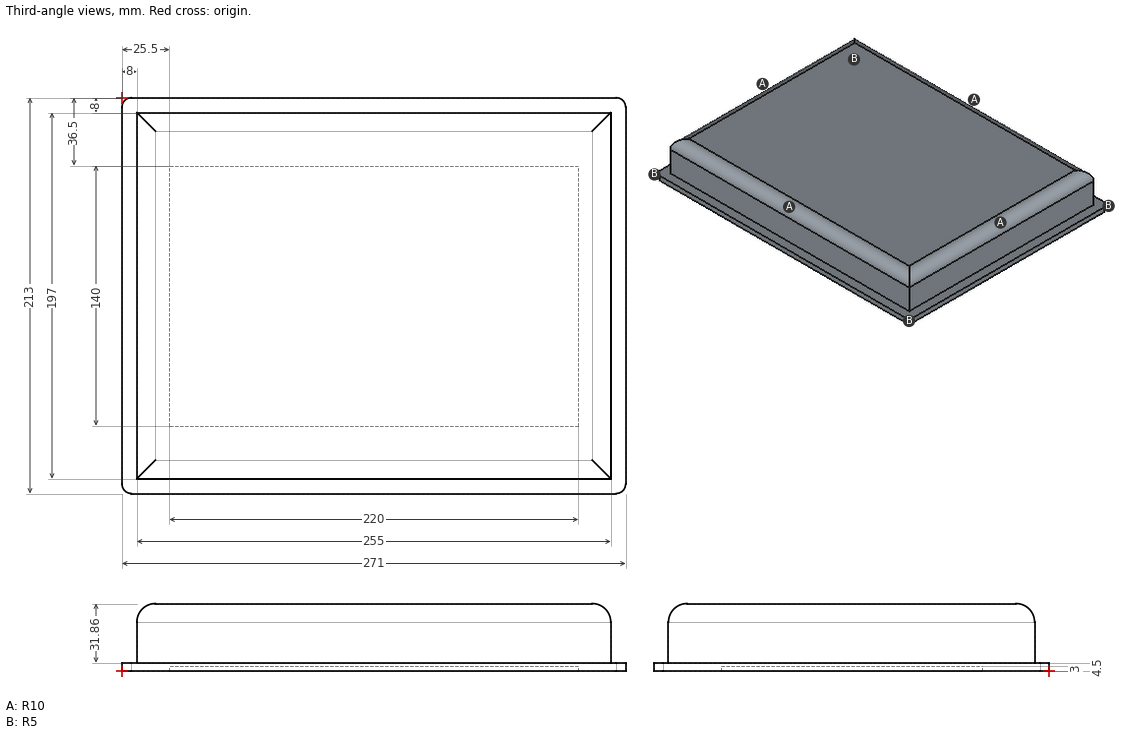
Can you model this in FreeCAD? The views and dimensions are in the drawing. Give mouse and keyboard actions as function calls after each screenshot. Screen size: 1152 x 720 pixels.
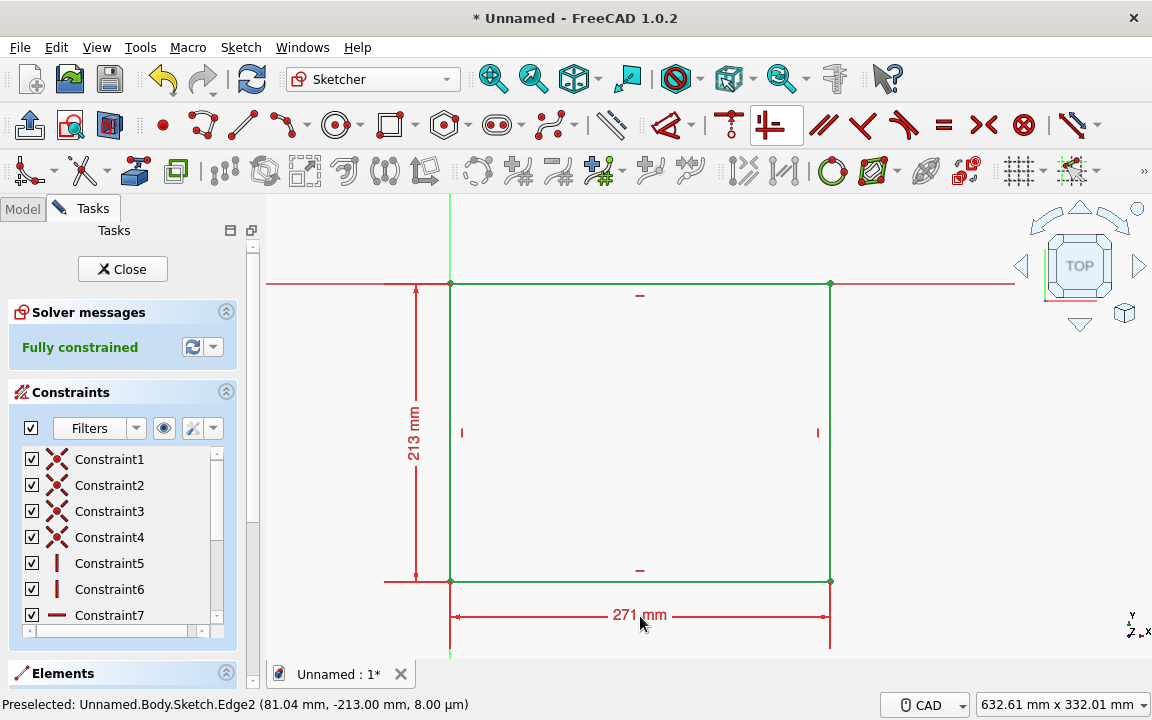
click(123, 269)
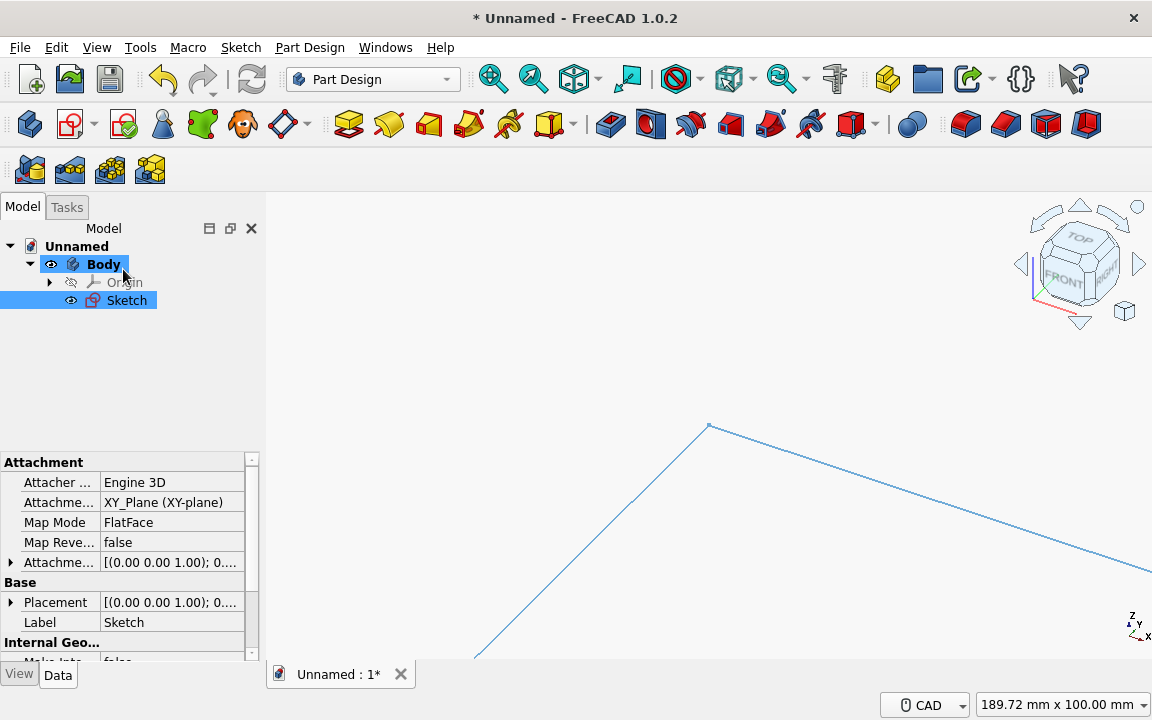
click(350, 124)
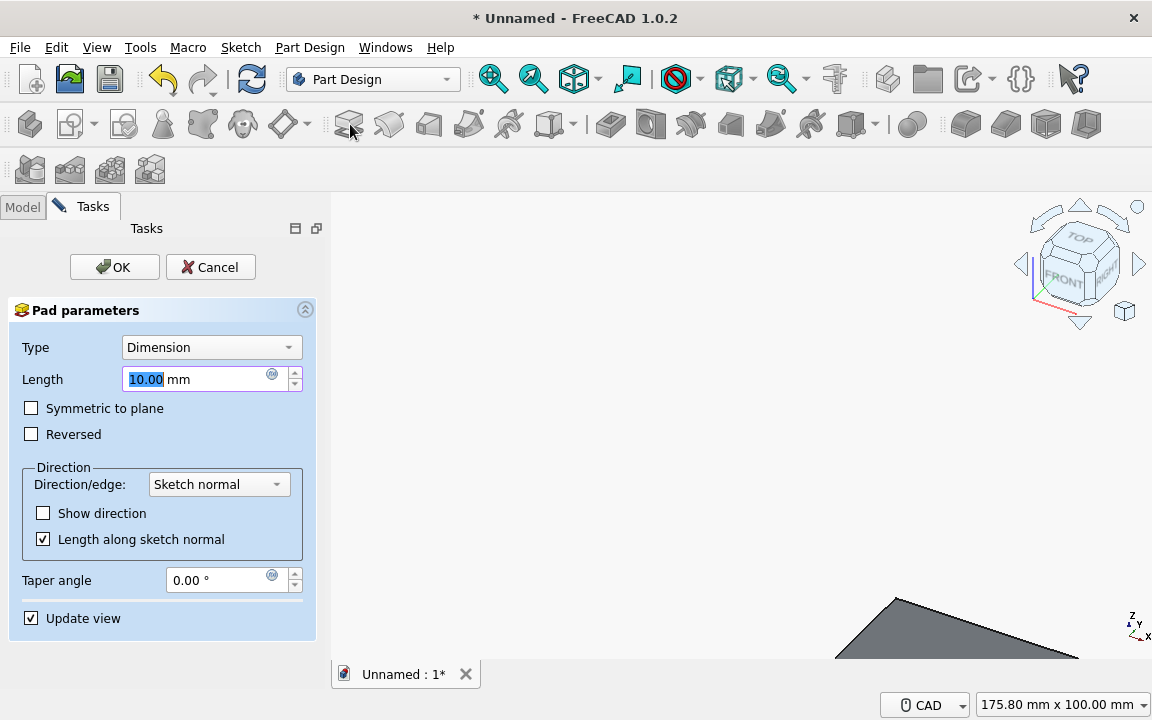
text(4.5)
key(Tab)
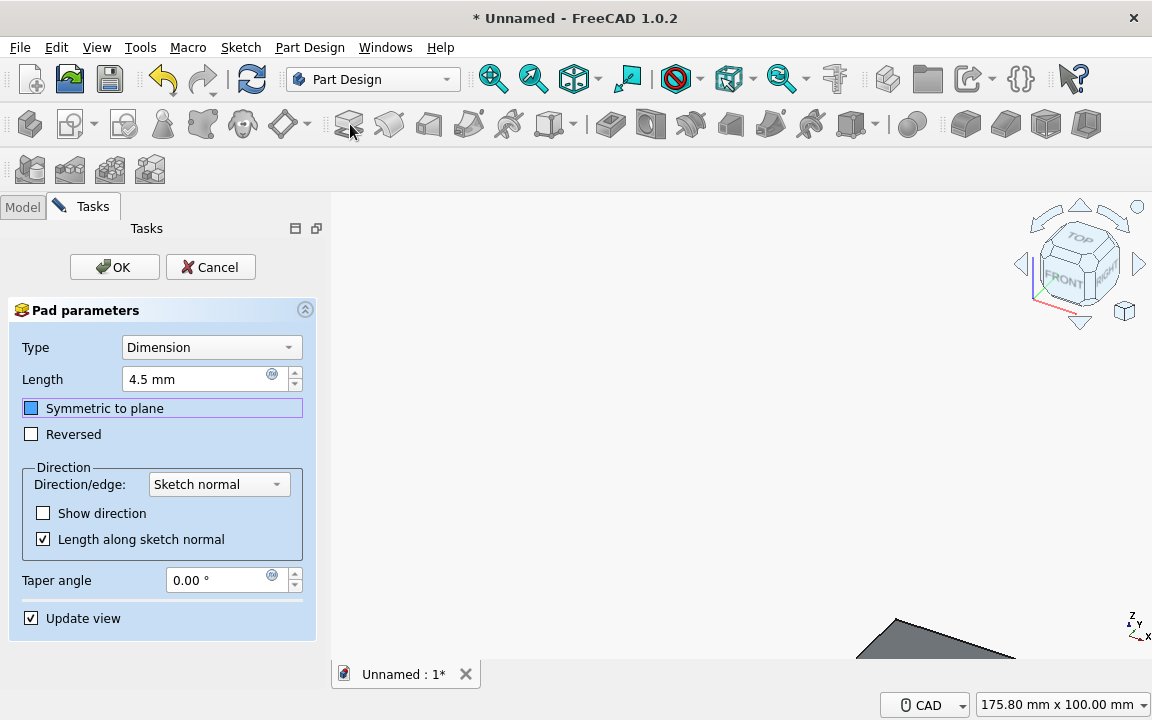
click(115, 267)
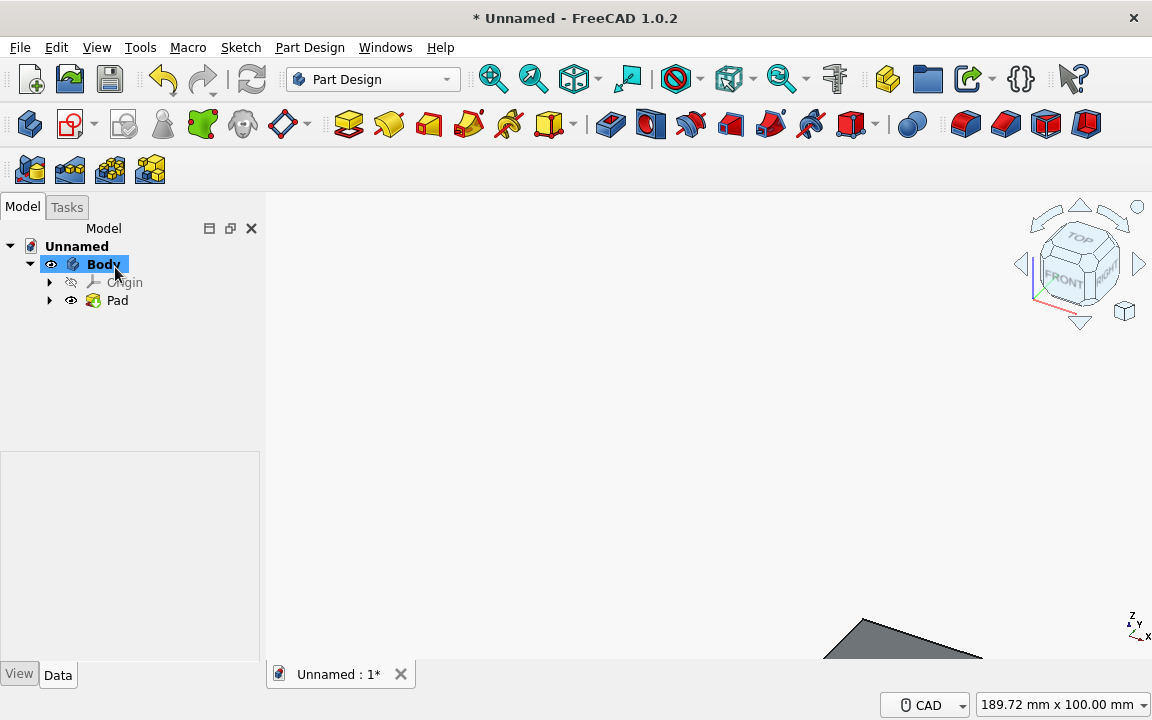
click(494, 80)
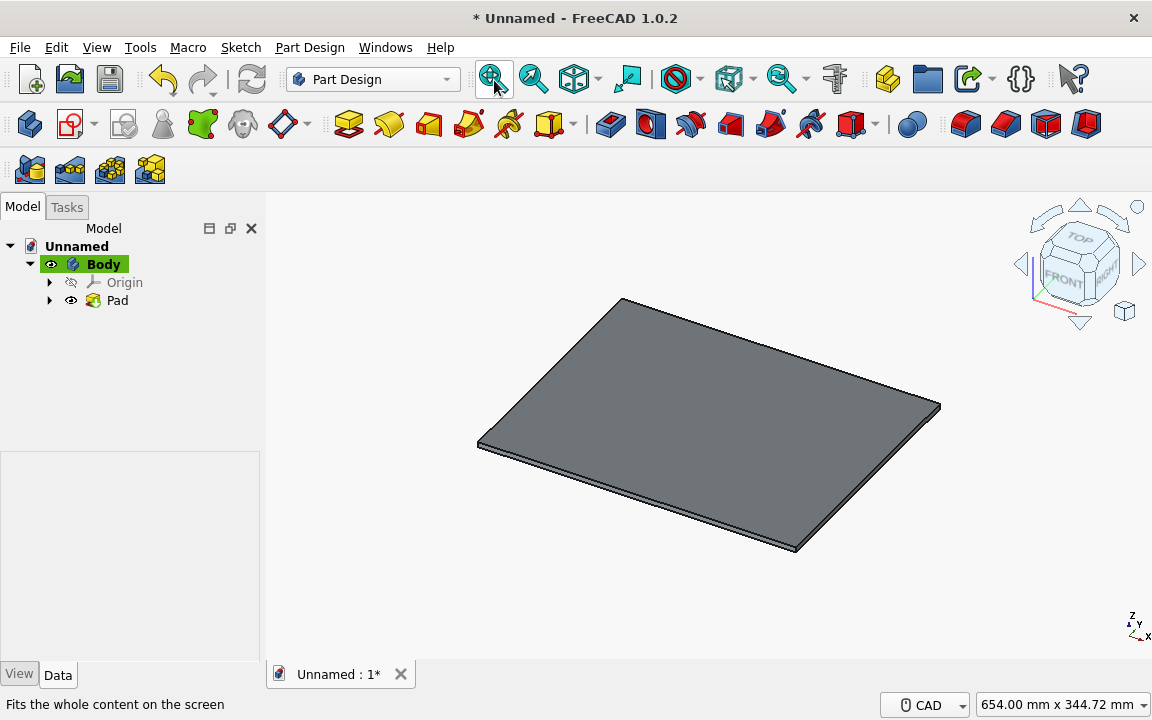
click(709, 422)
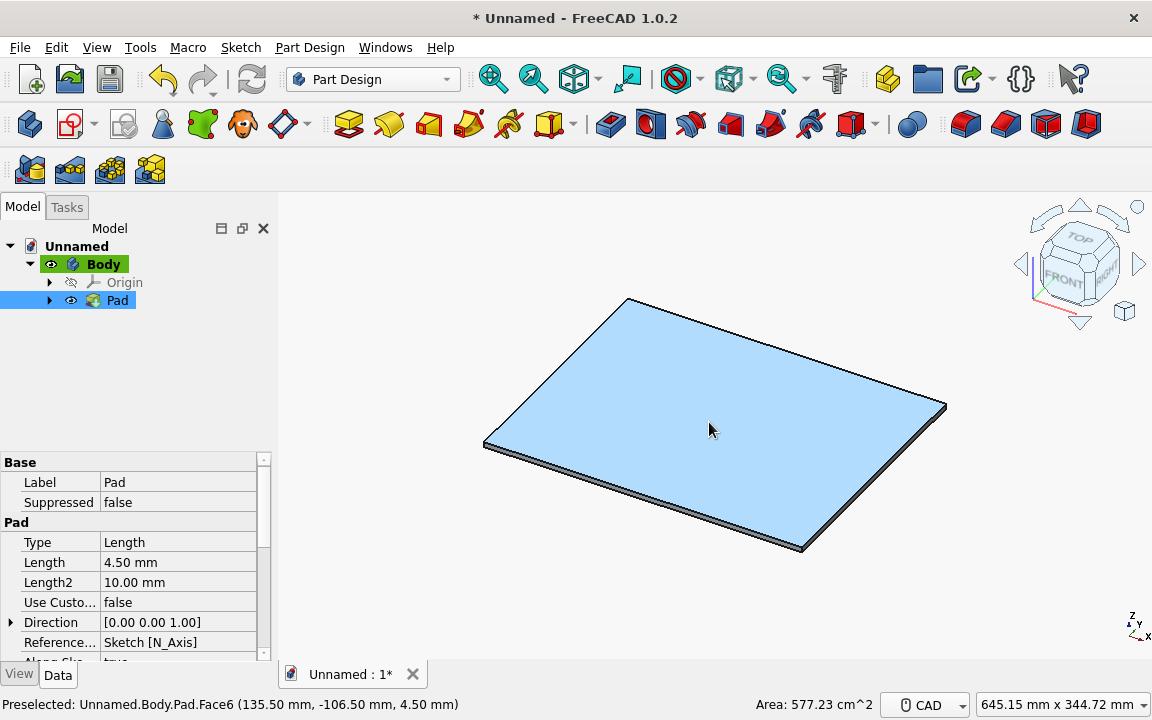
click(70, 124)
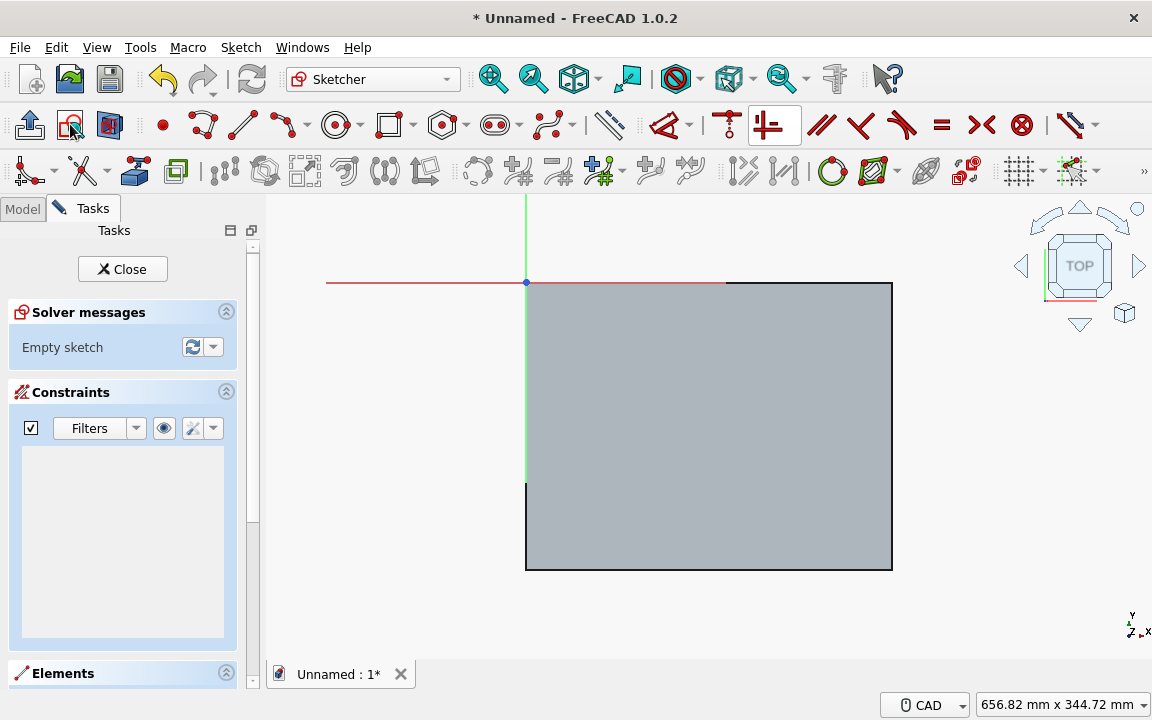
click(390, 126)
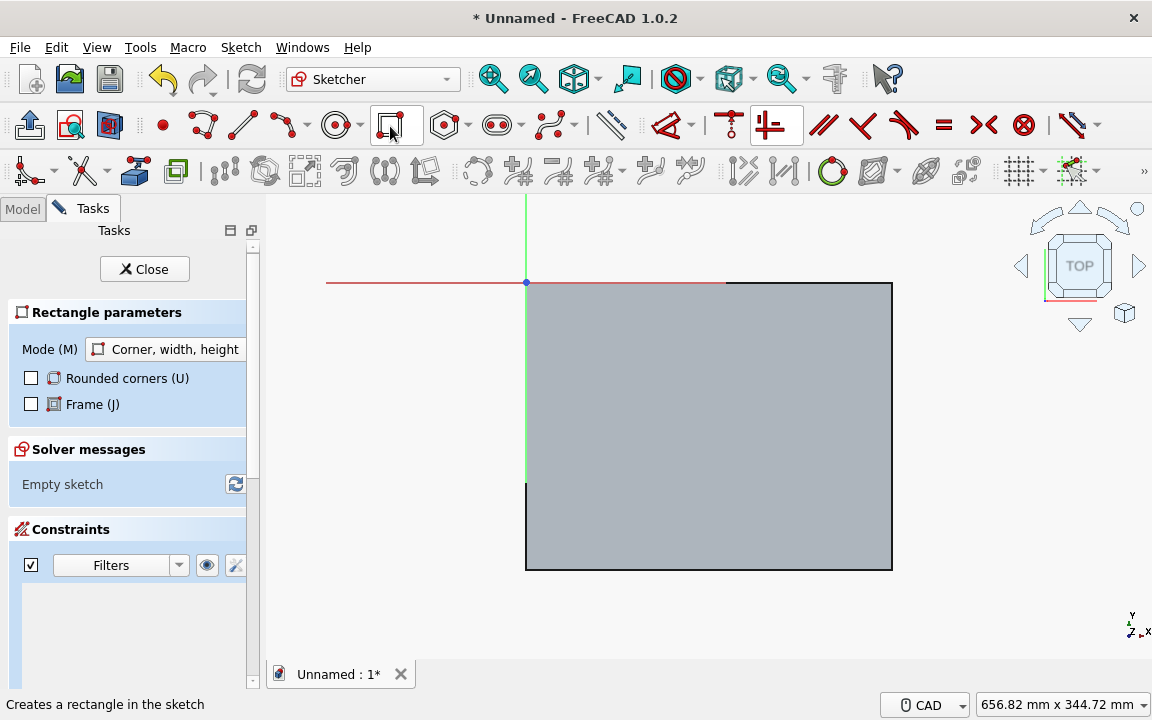
scroll(537, 294, up, 2)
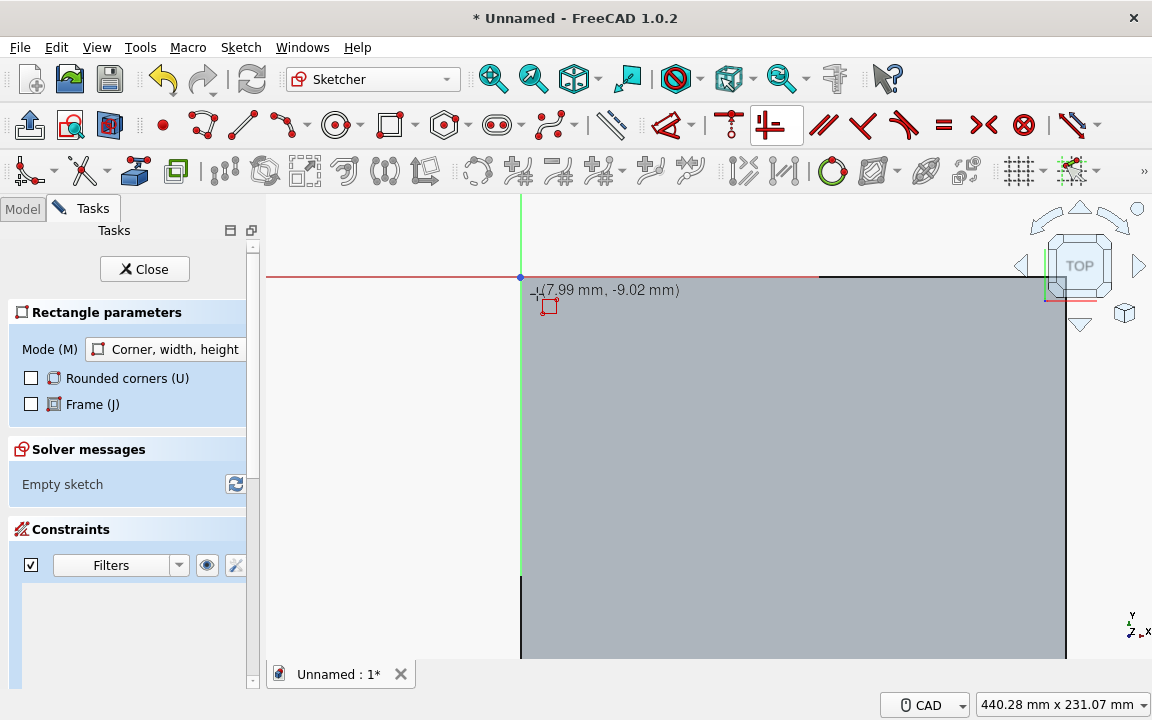
click(537, 293)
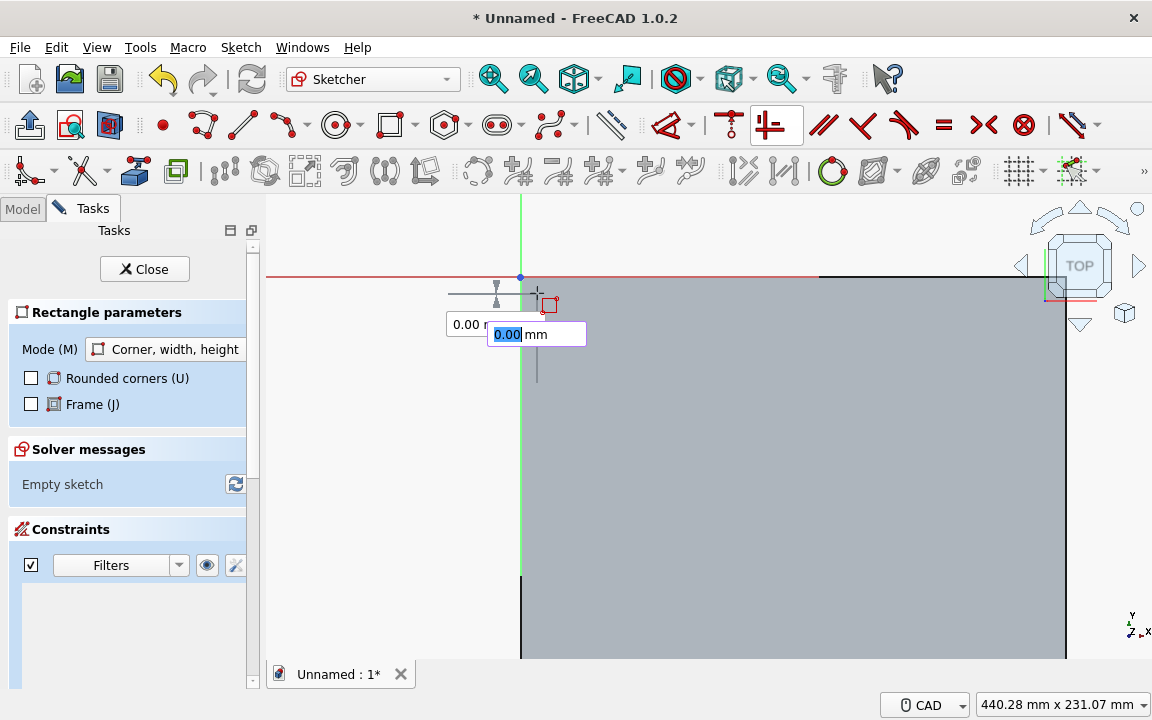
scroll(346, 311, down, 2)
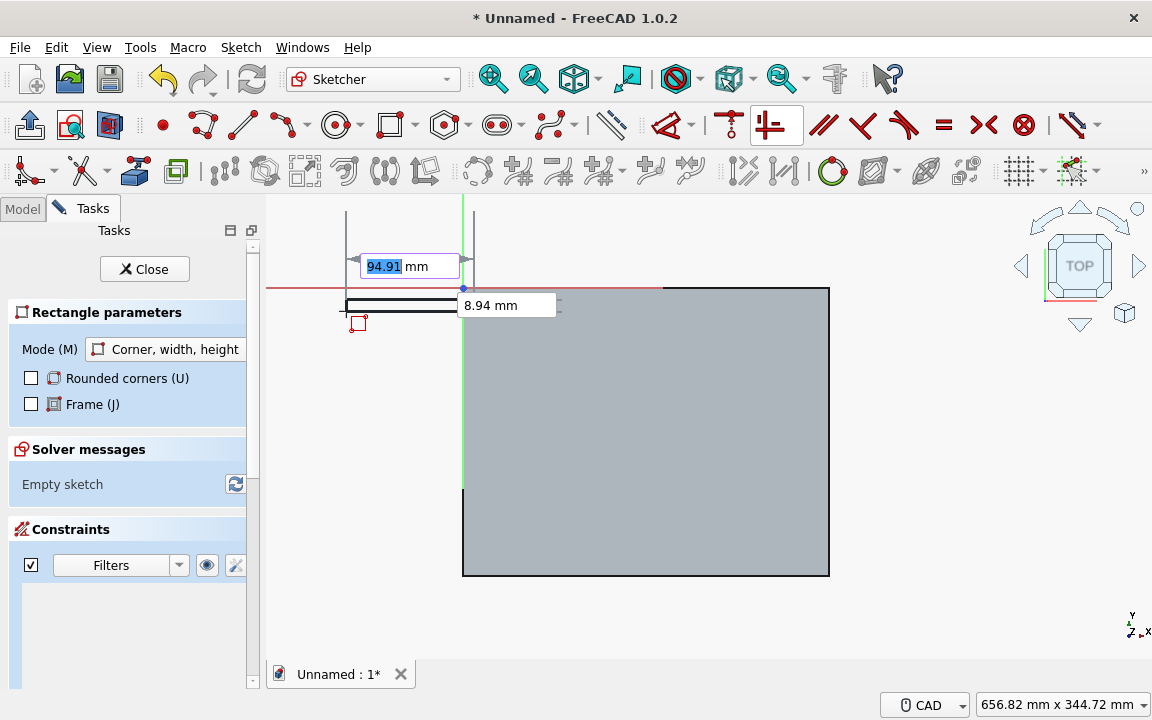
click(818, 565)
key(Escape)